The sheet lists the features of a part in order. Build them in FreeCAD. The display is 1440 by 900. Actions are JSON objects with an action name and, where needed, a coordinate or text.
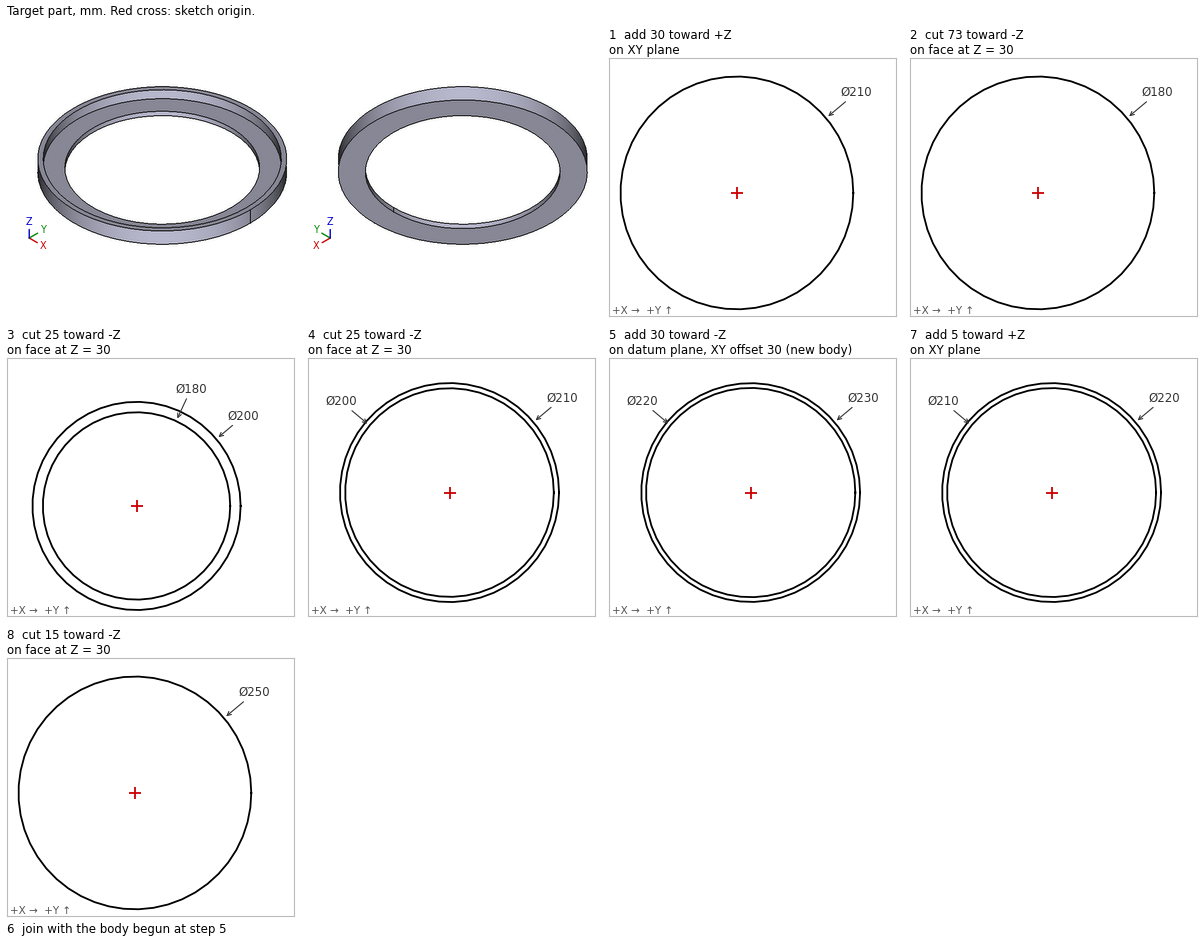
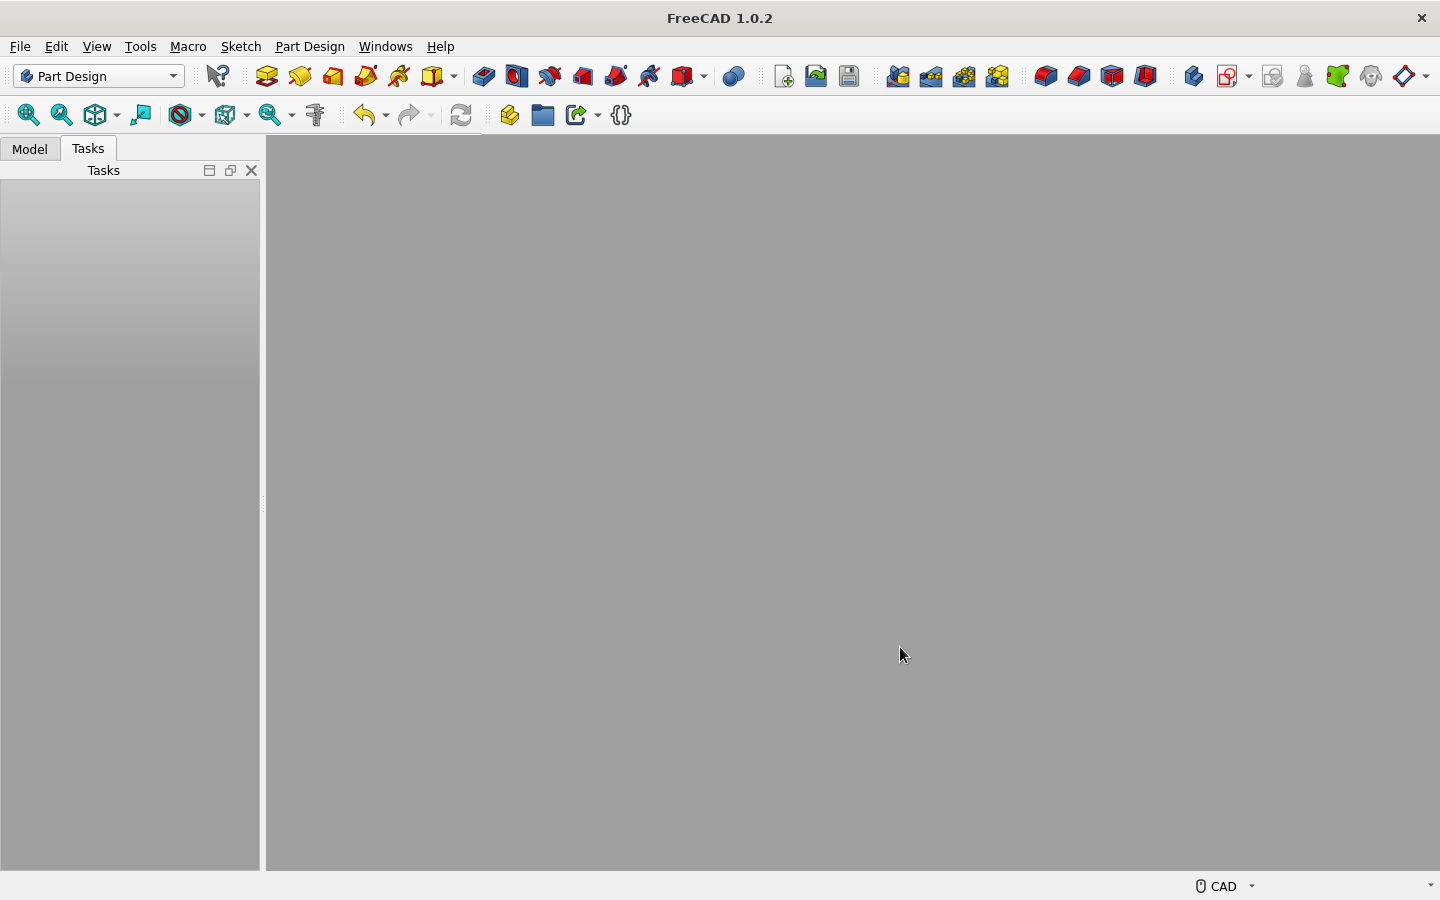
{"action": "left_click", "coordinate": [783, 76]}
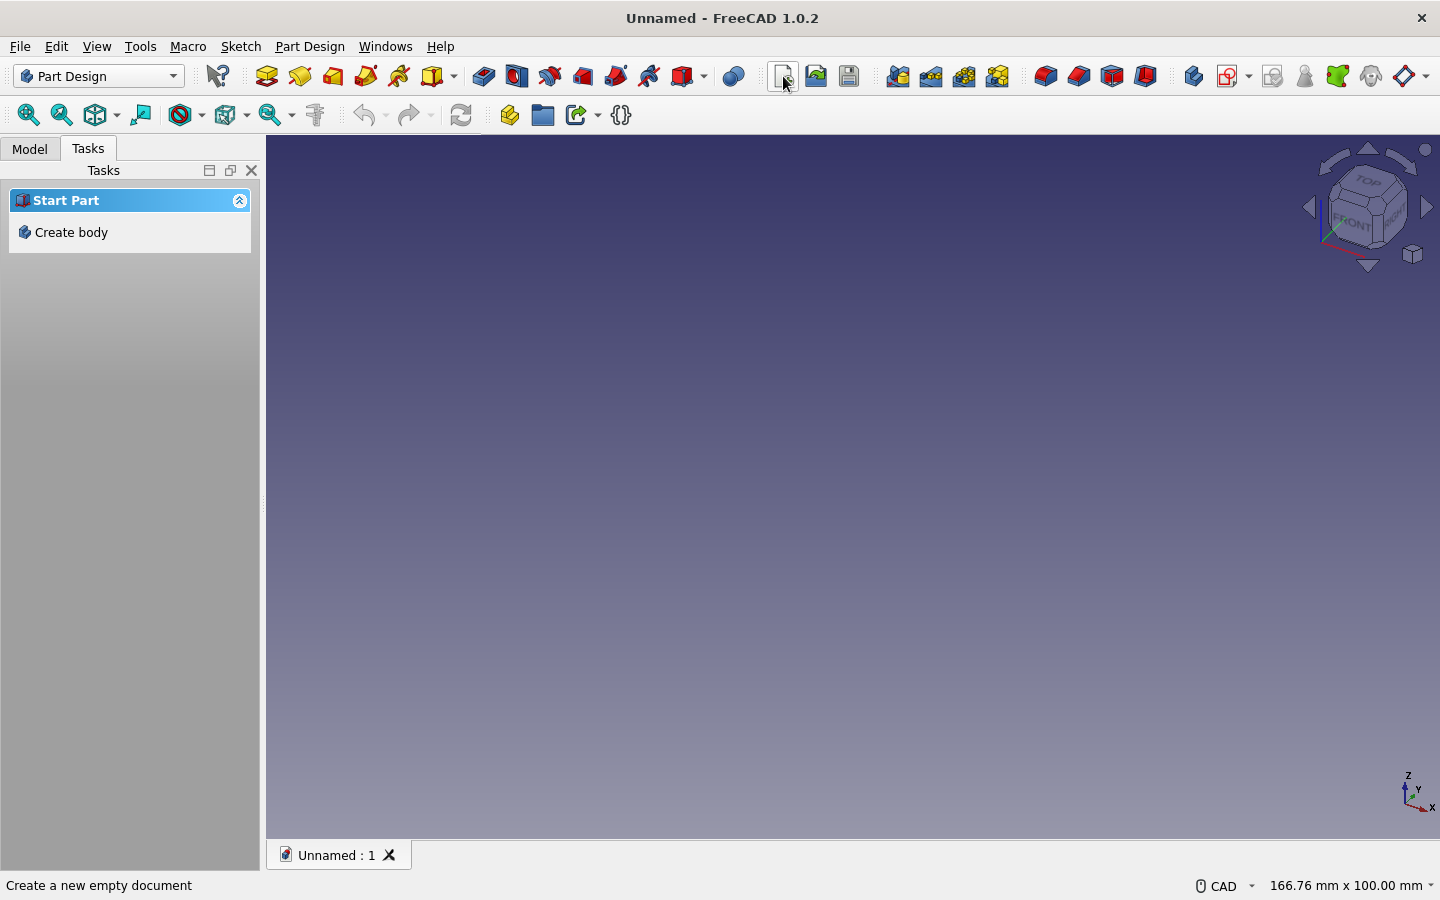
{"action": "left_click", "coordinate": [1226, 76]}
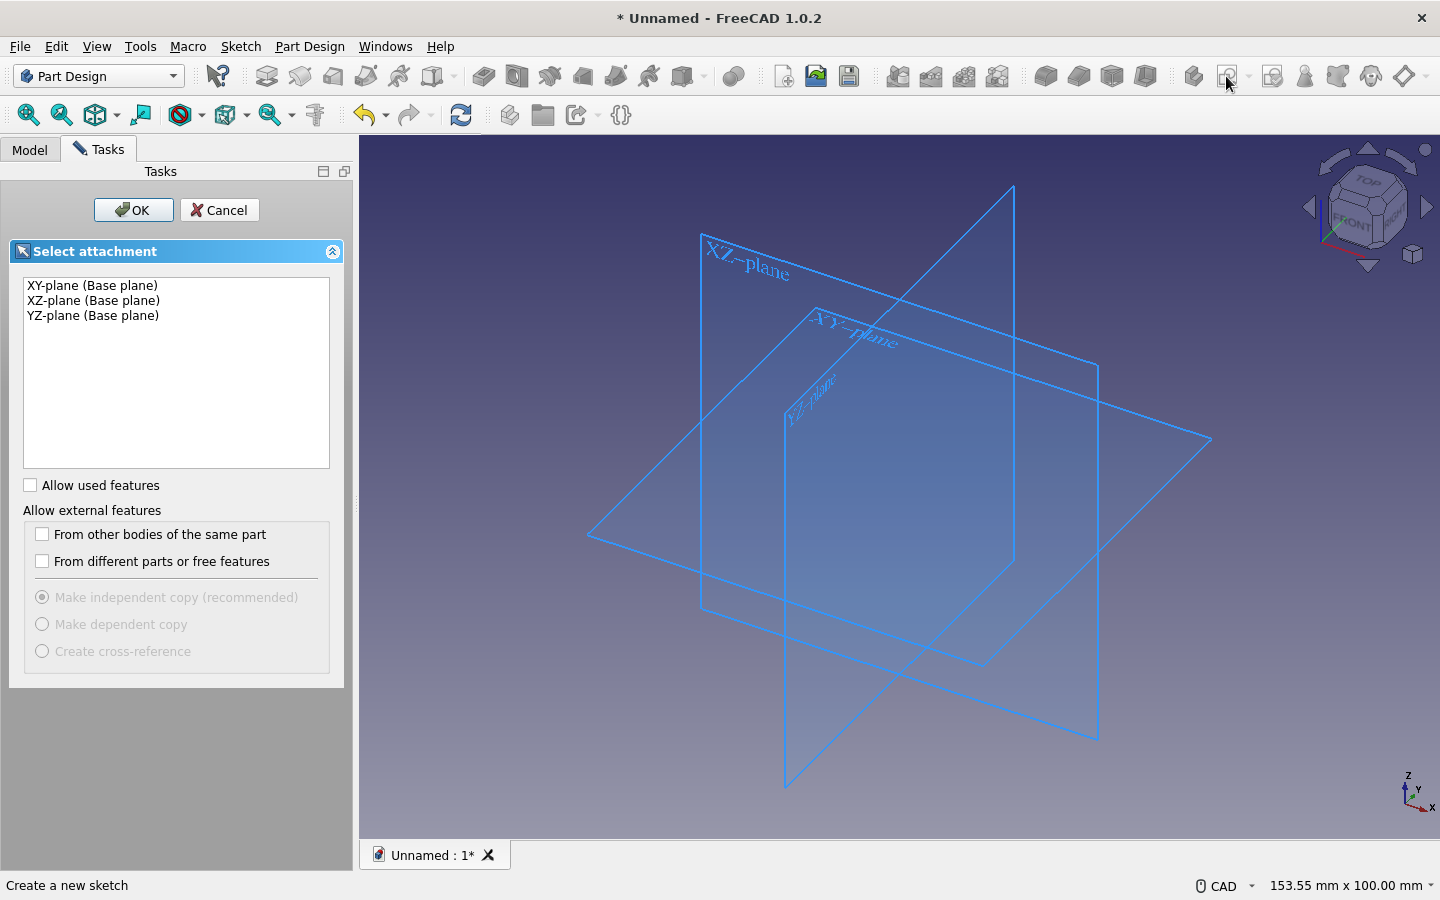
{"action": "left_click", "coordinate": [84, 286]}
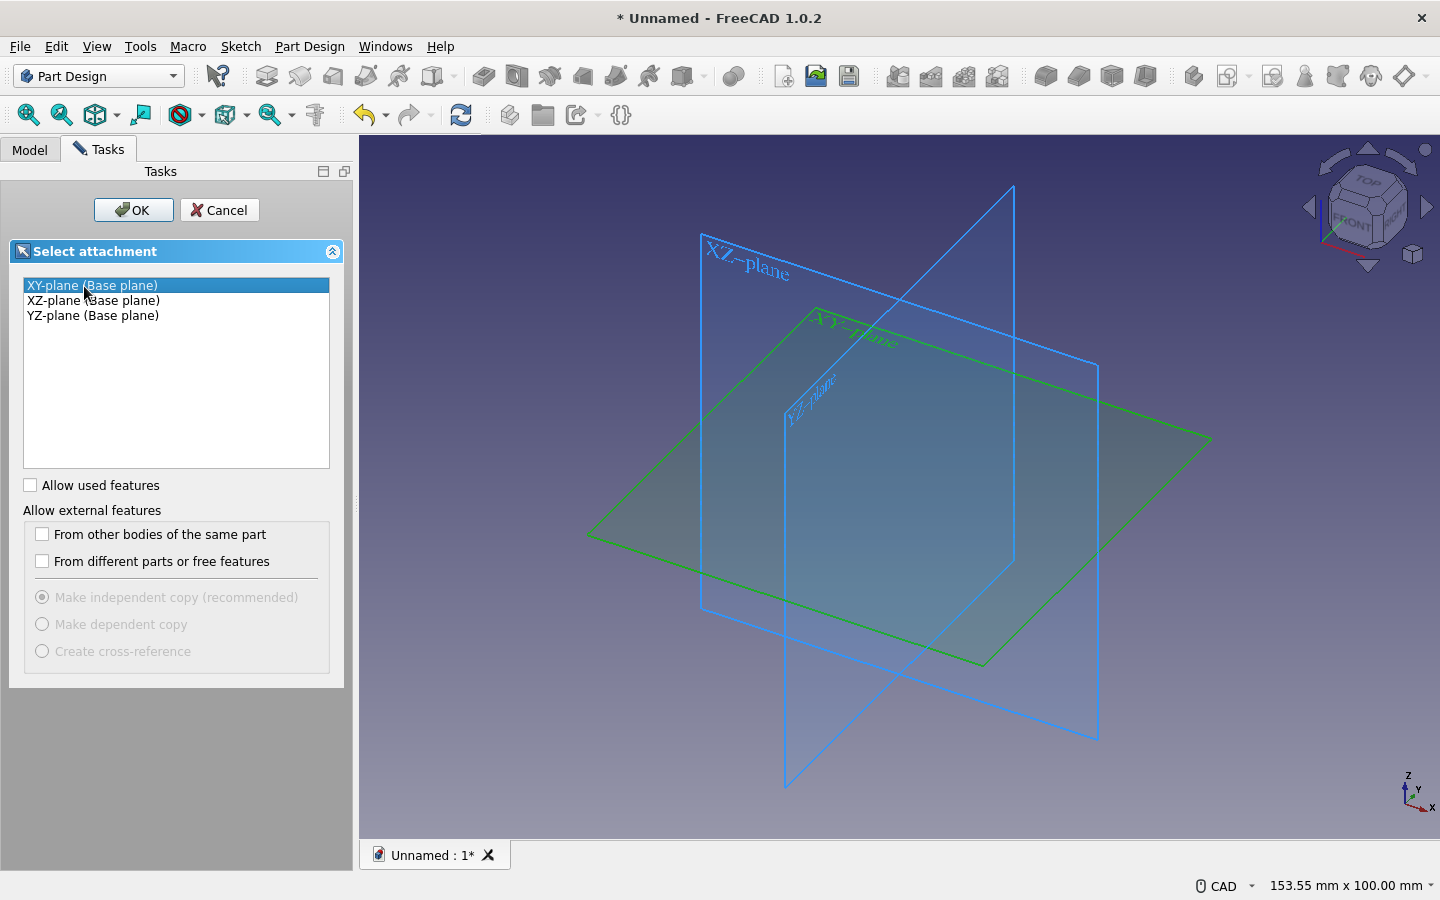
{"action": "left_click", "coordinate": [134, 210]}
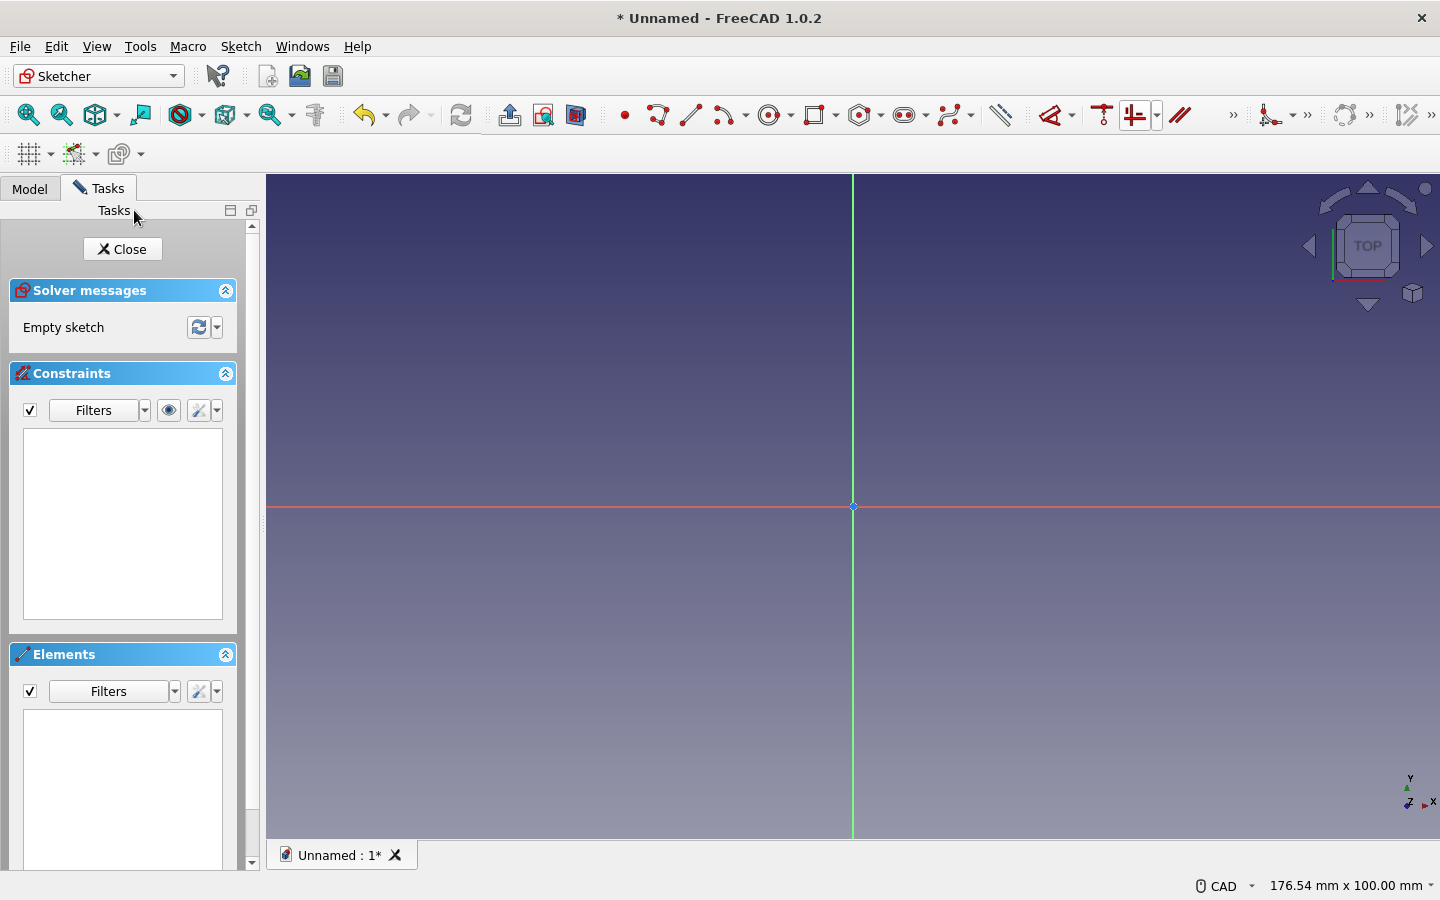
{"action": "scroll", "coordinate": [755, 506], "scroll_direction": "down", "scroll_amount": 6}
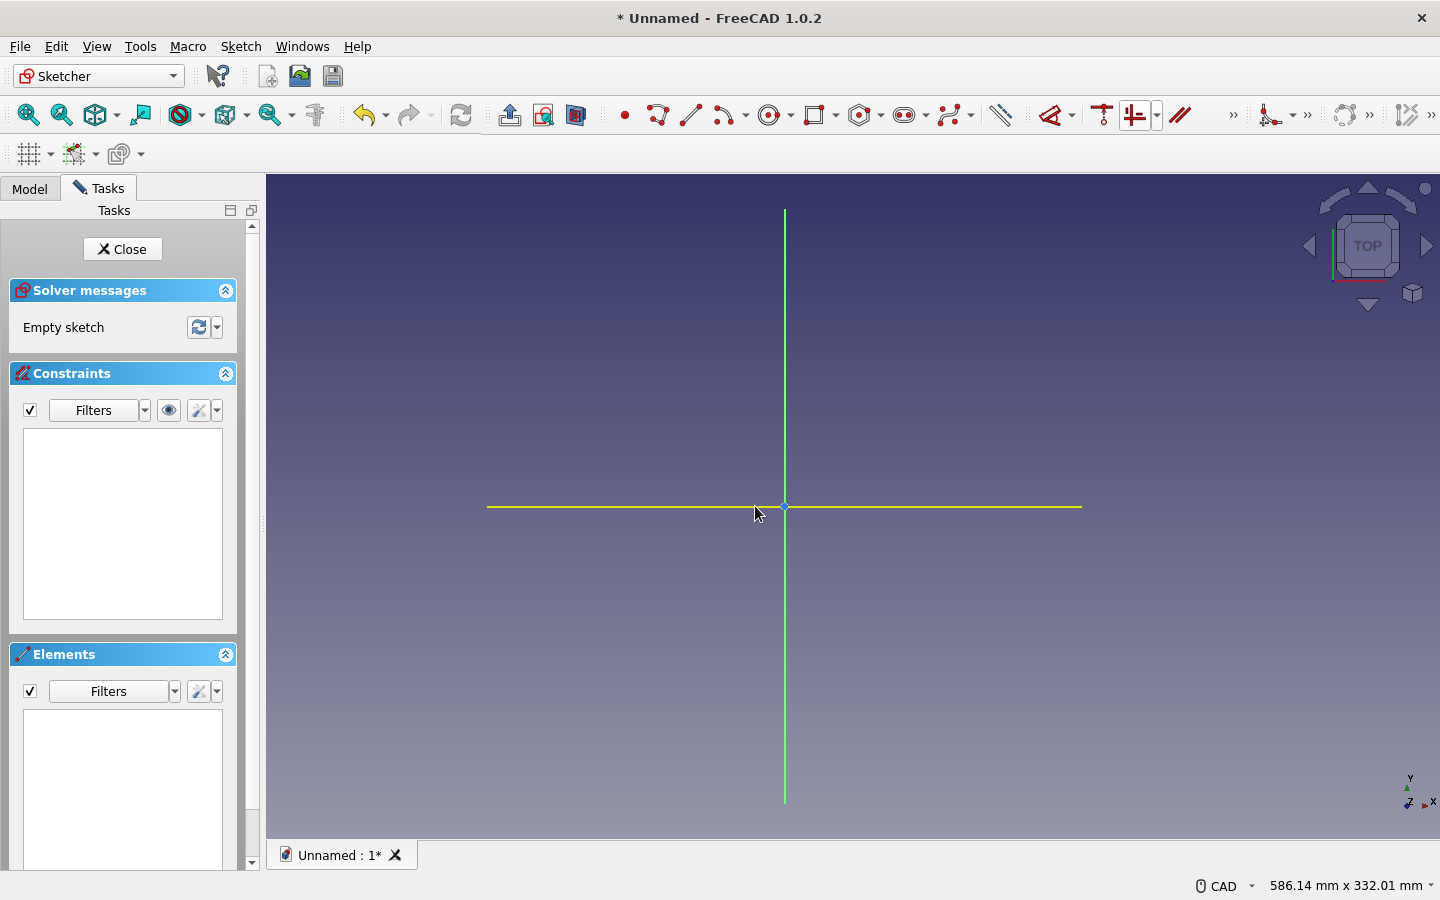
{"action": "left_click", "coordinate": [768, 116]}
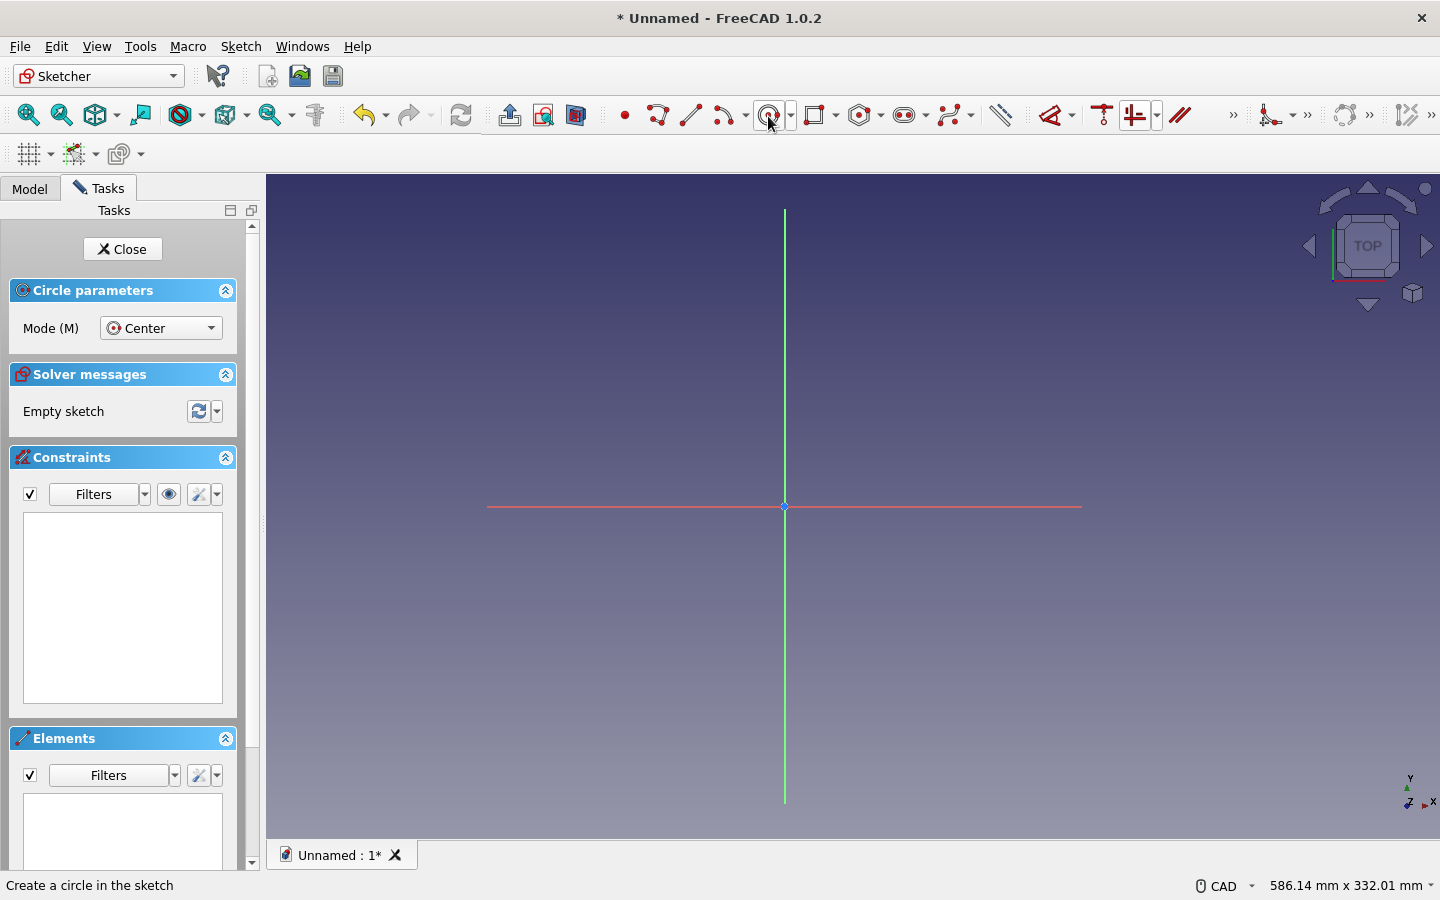
{"action": "left_click", "coordinate": [785, 506]}
{"action": "mouse_move", "coordinate": [934, 358]}